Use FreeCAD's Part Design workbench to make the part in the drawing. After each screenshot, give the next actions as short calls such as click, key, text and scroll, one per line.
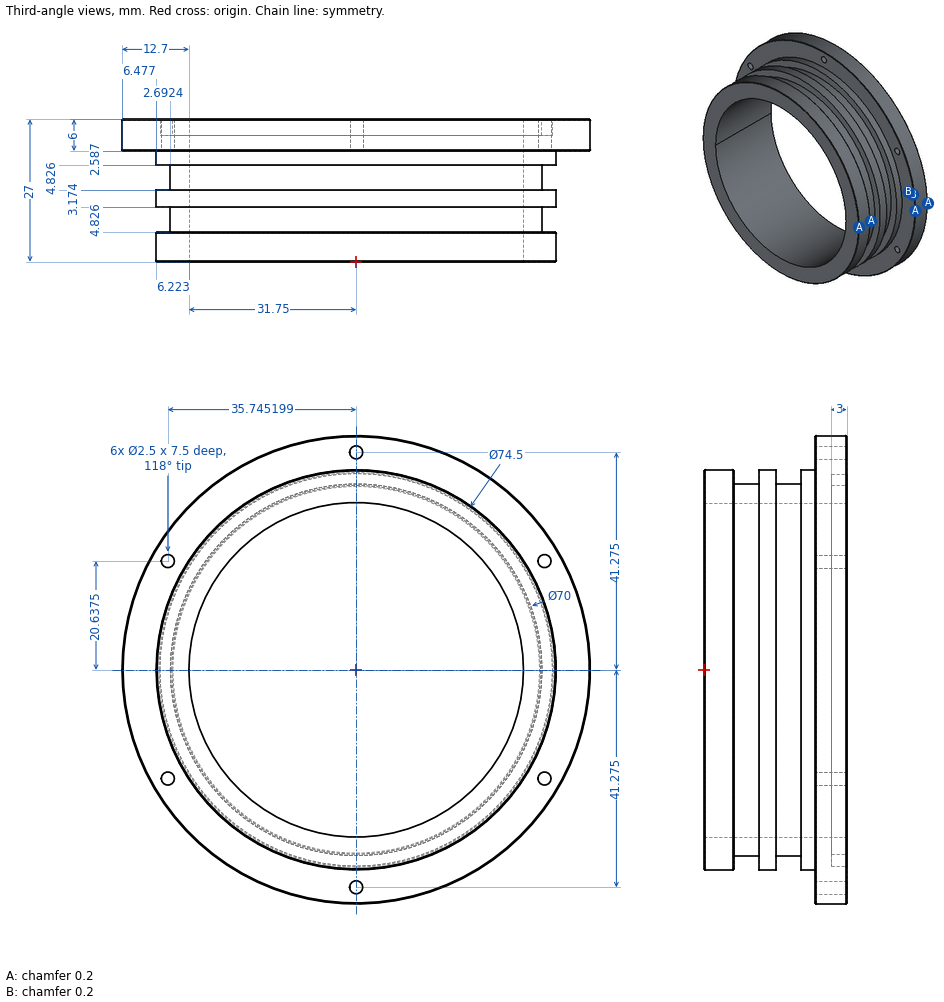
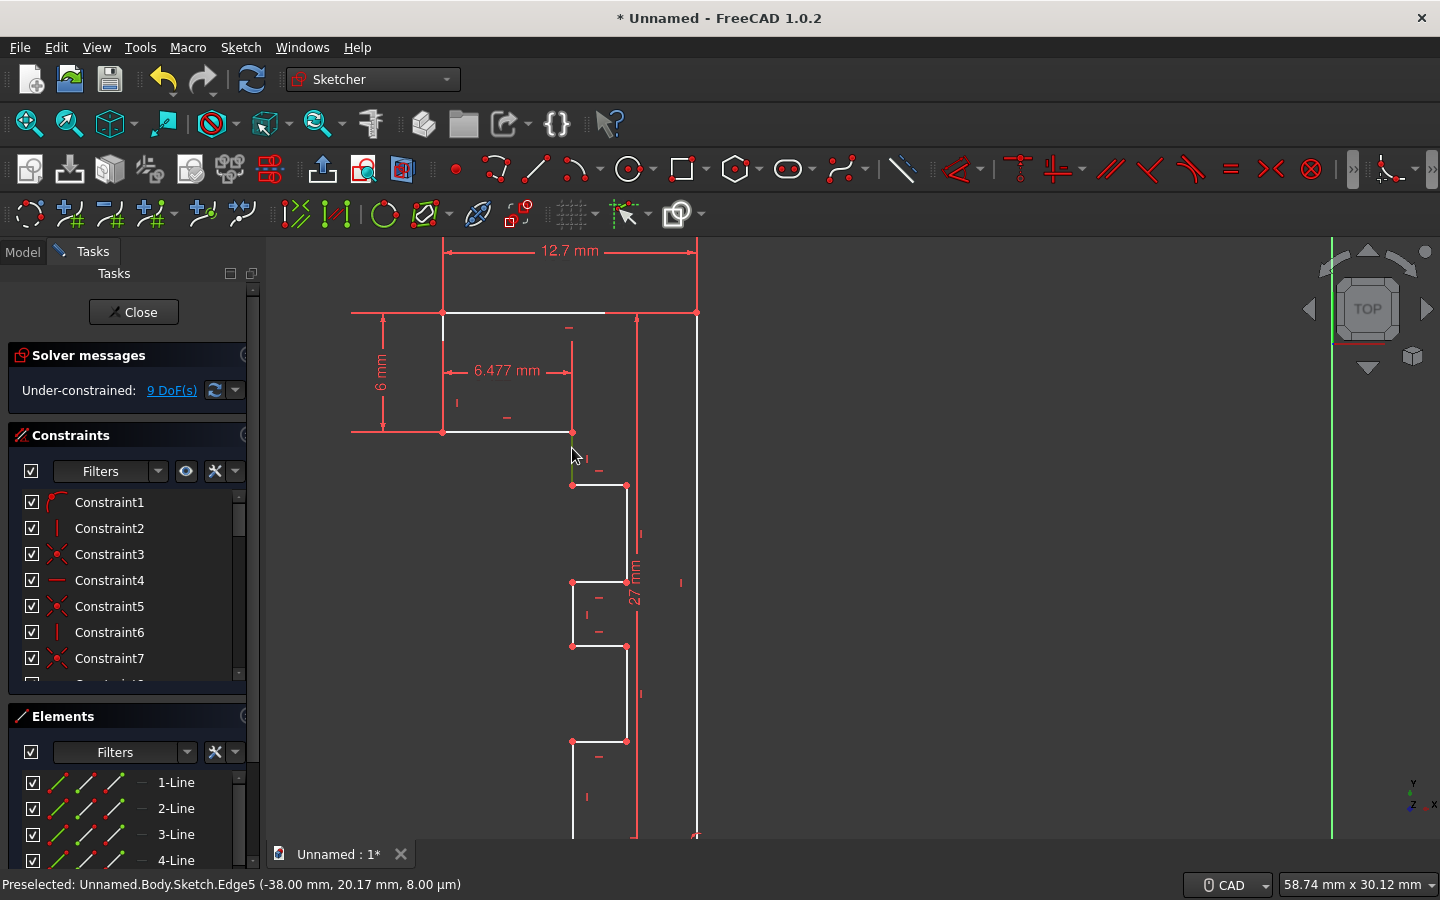
key(i)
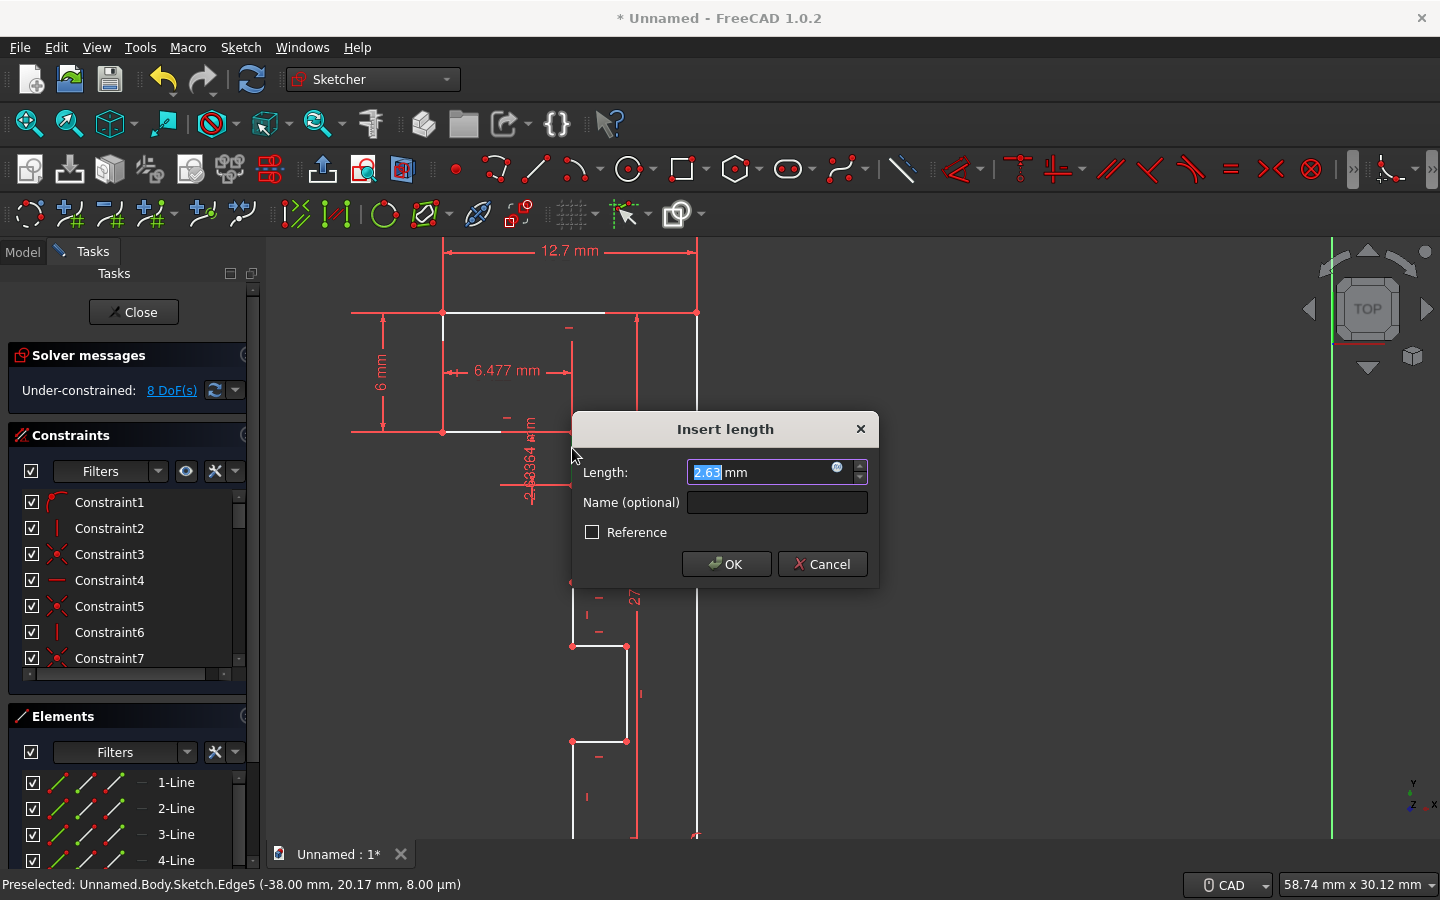
text(2.587)
key(Return)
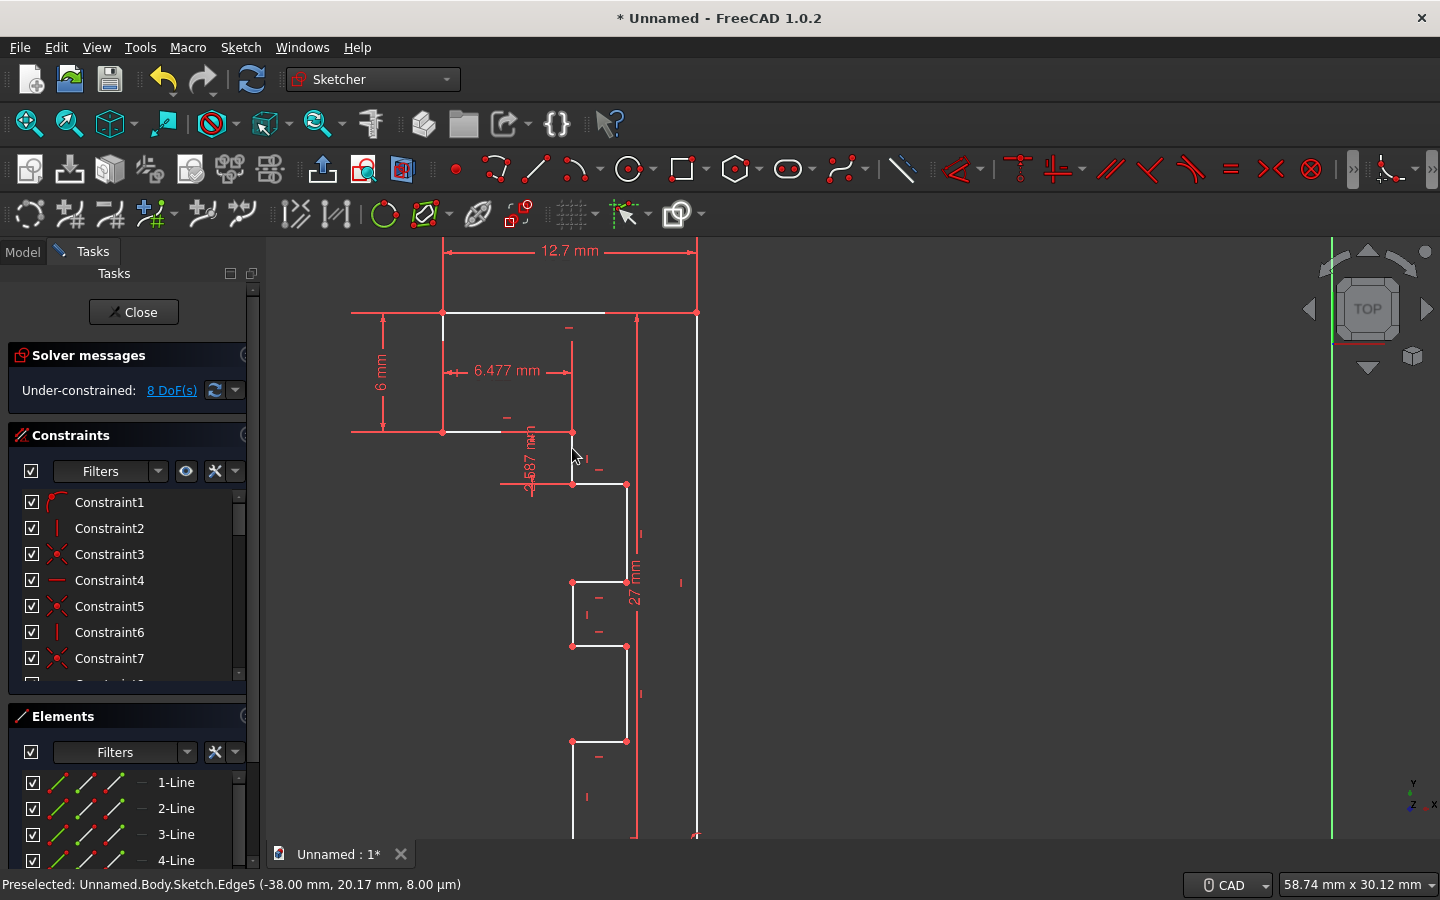
click(627, 514)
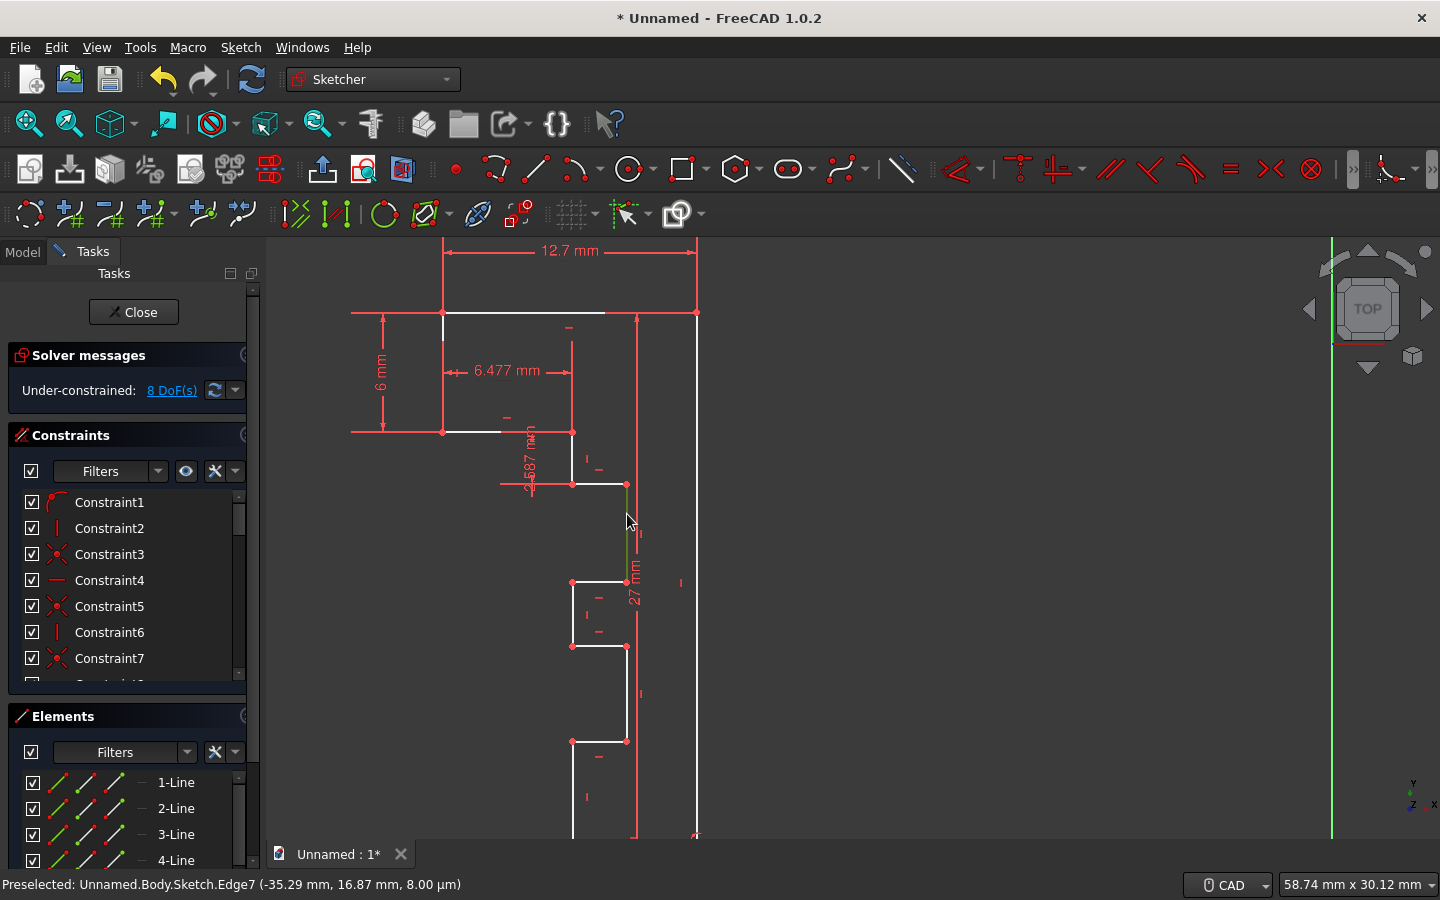
key(i)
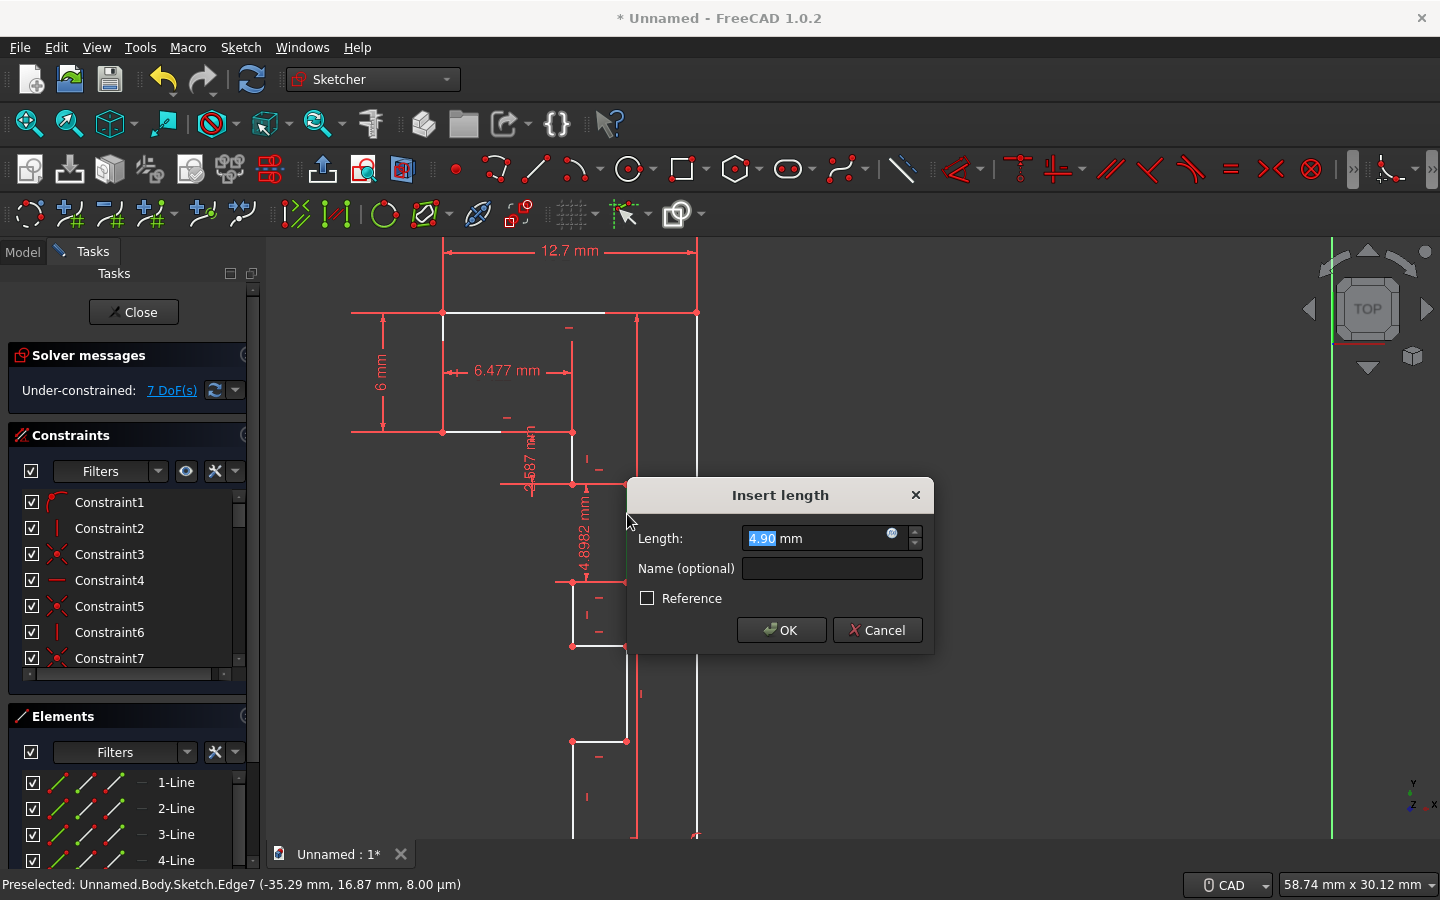
text(4.826)
key(Return)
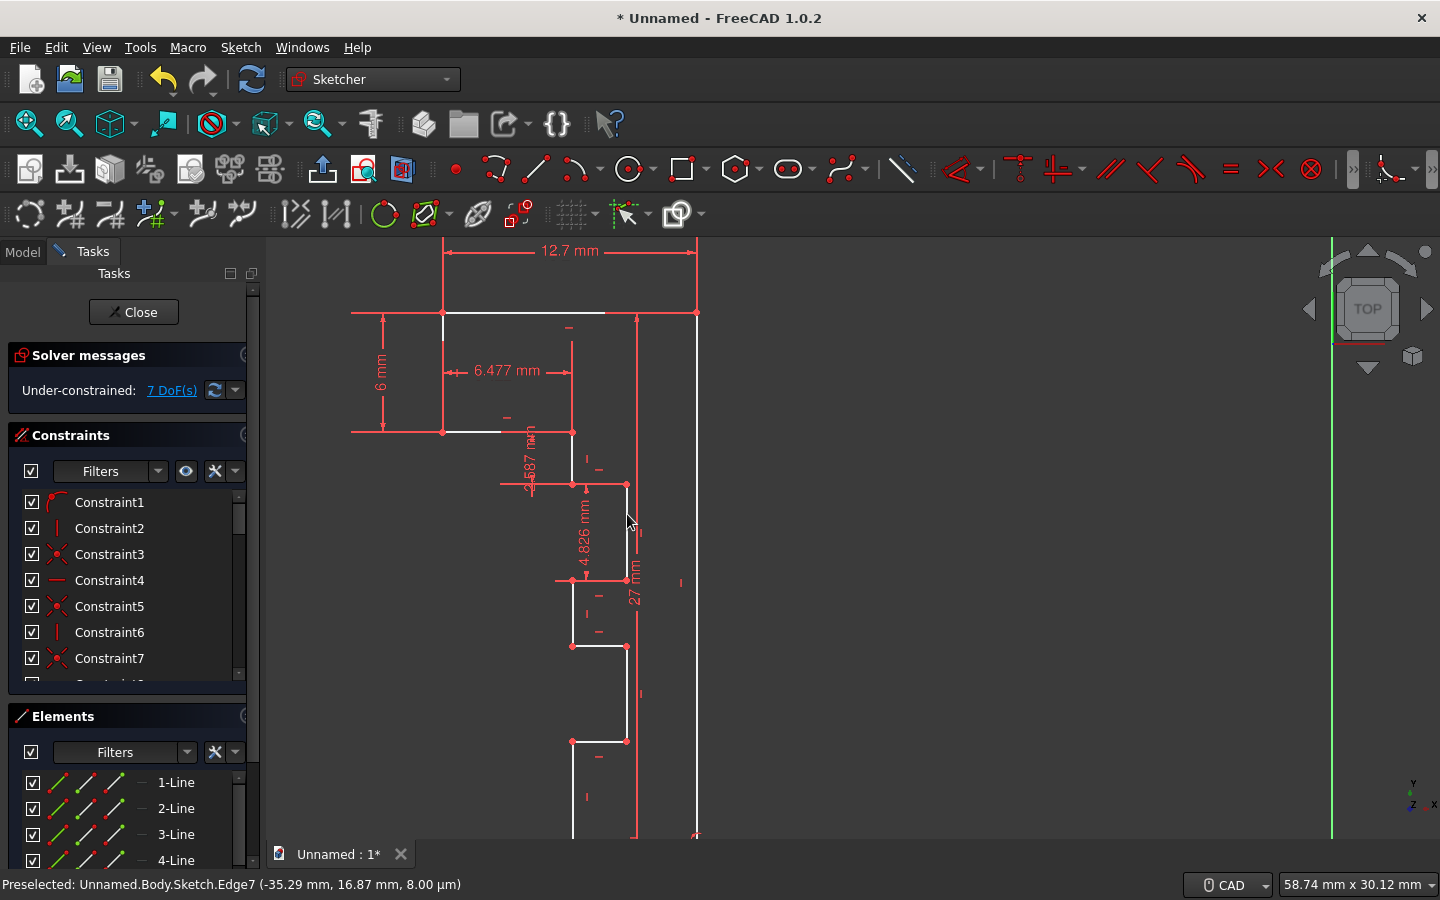
click(573, 600)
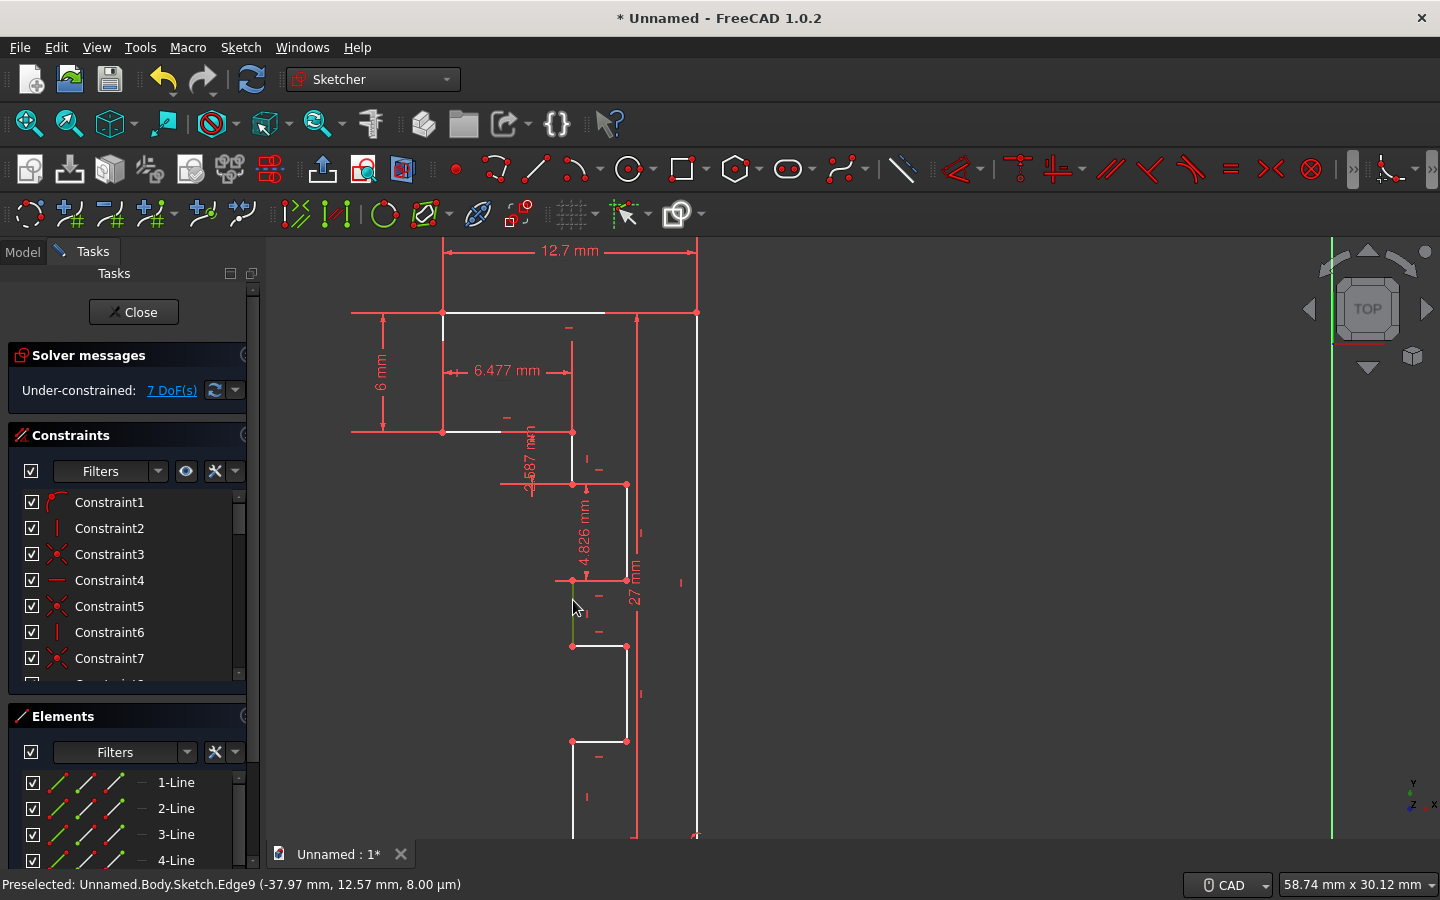
click(982, 170)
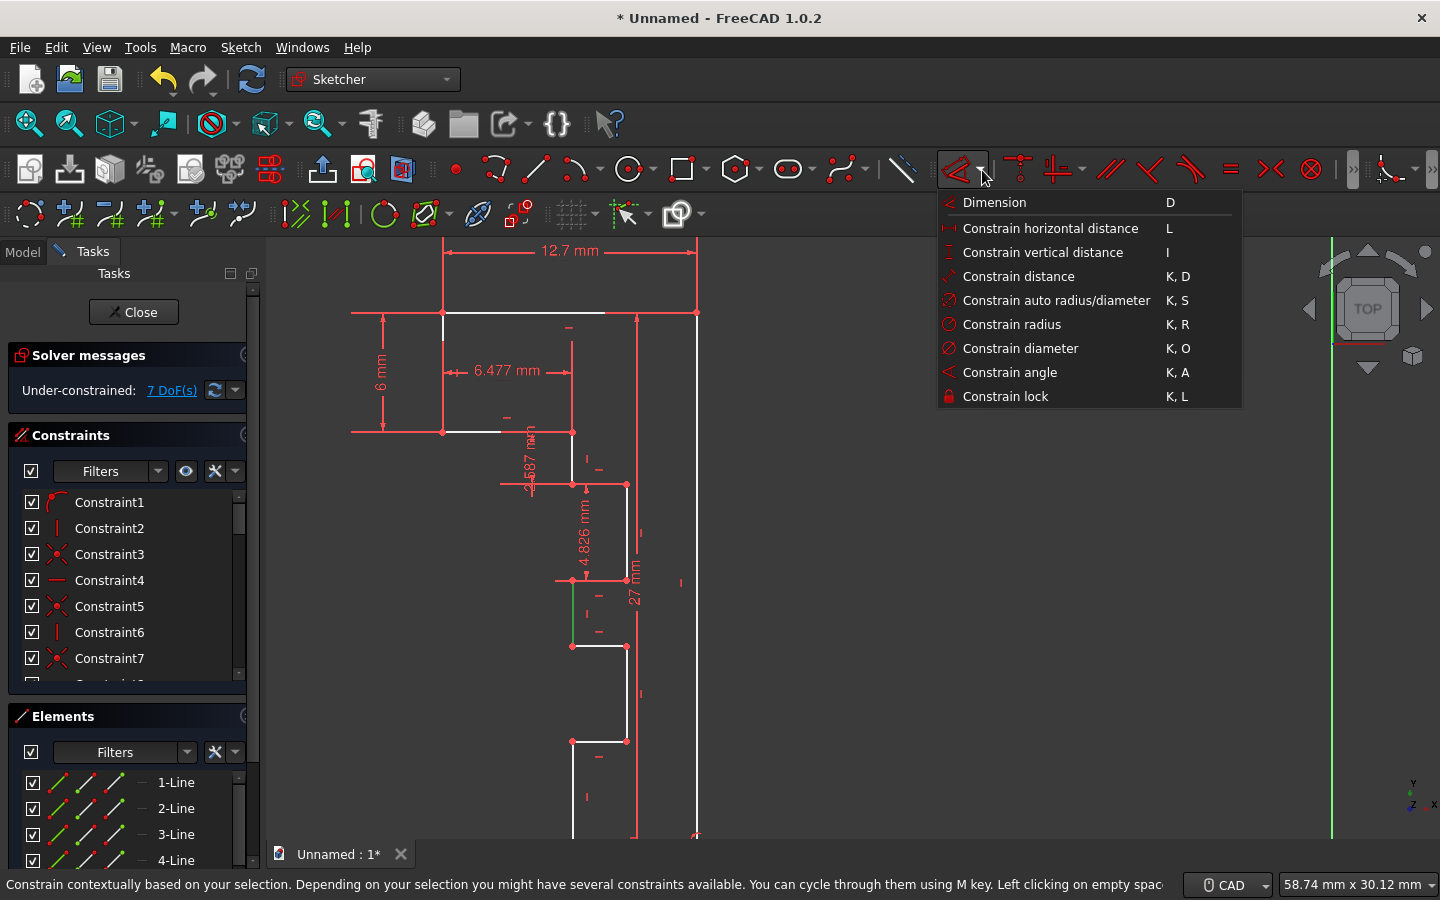
click(1090, 252)